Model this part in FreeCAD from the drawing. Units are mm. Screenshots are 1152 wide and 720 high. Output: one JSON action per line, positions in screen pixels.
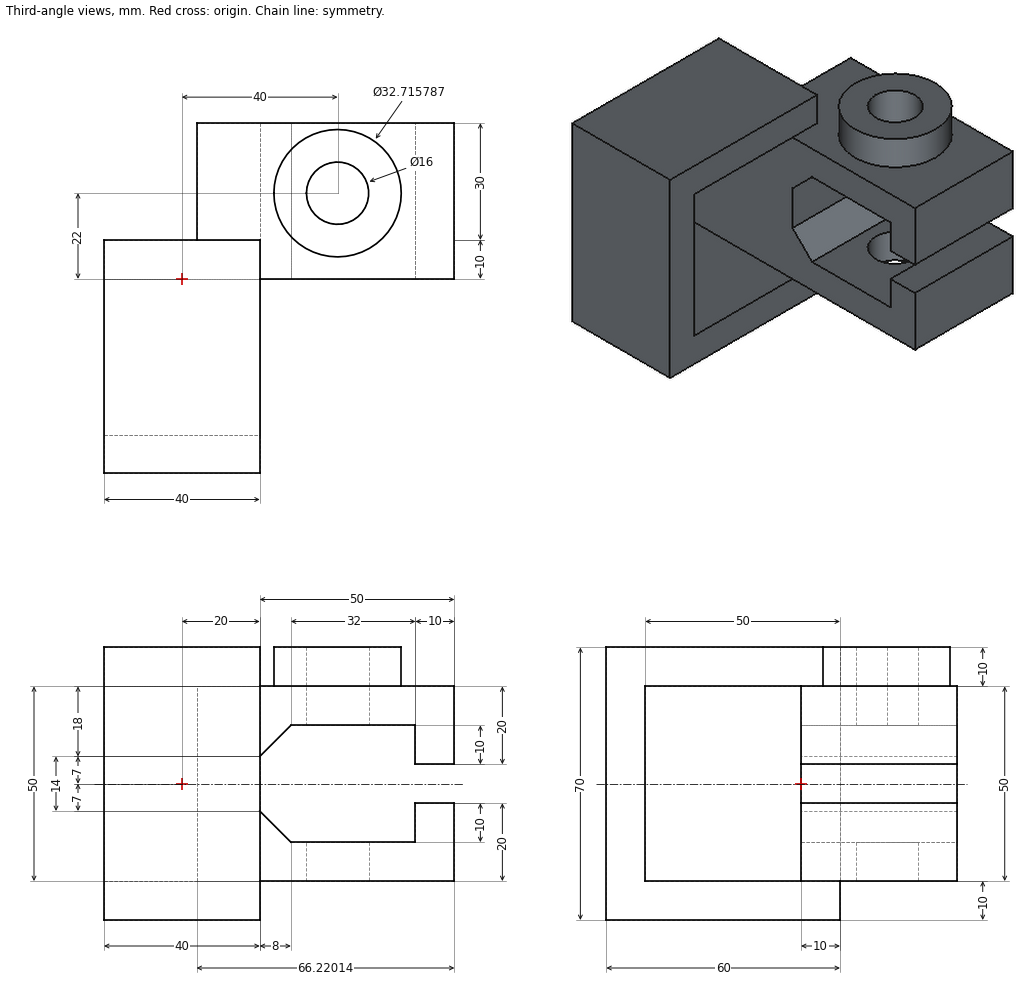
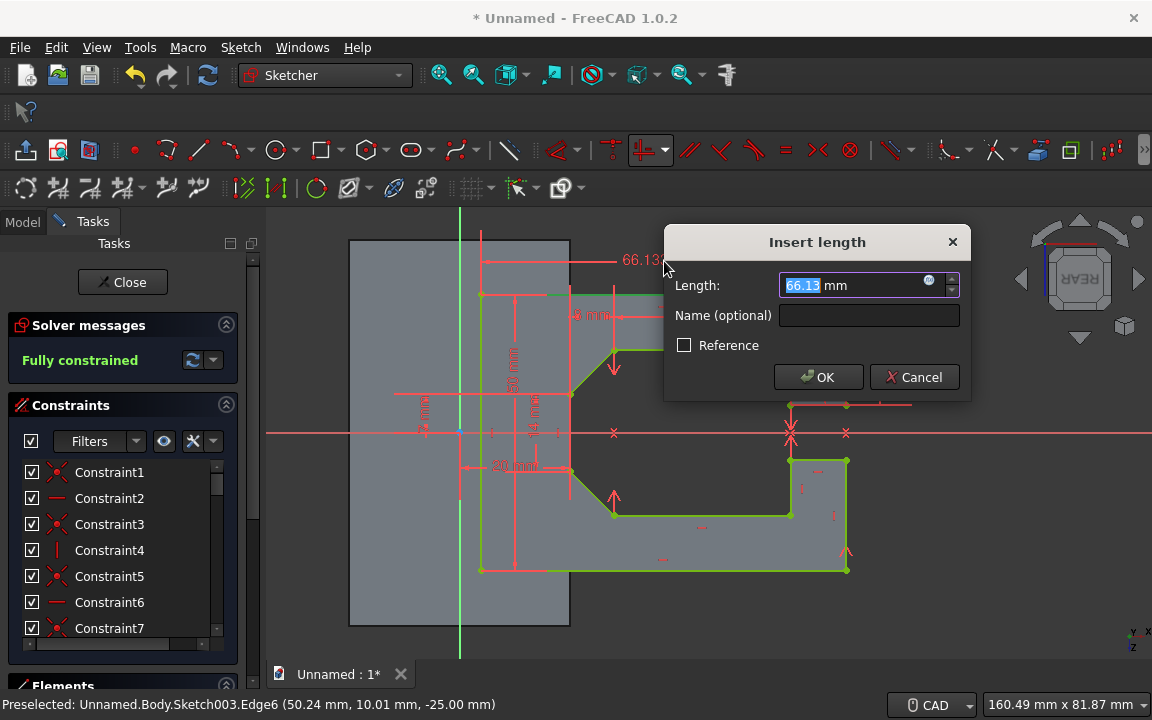
{"action": "type", "text": "66.22014"}
{"action": "key", "text": "Return"}
{"action": "key", "text": "Escape"}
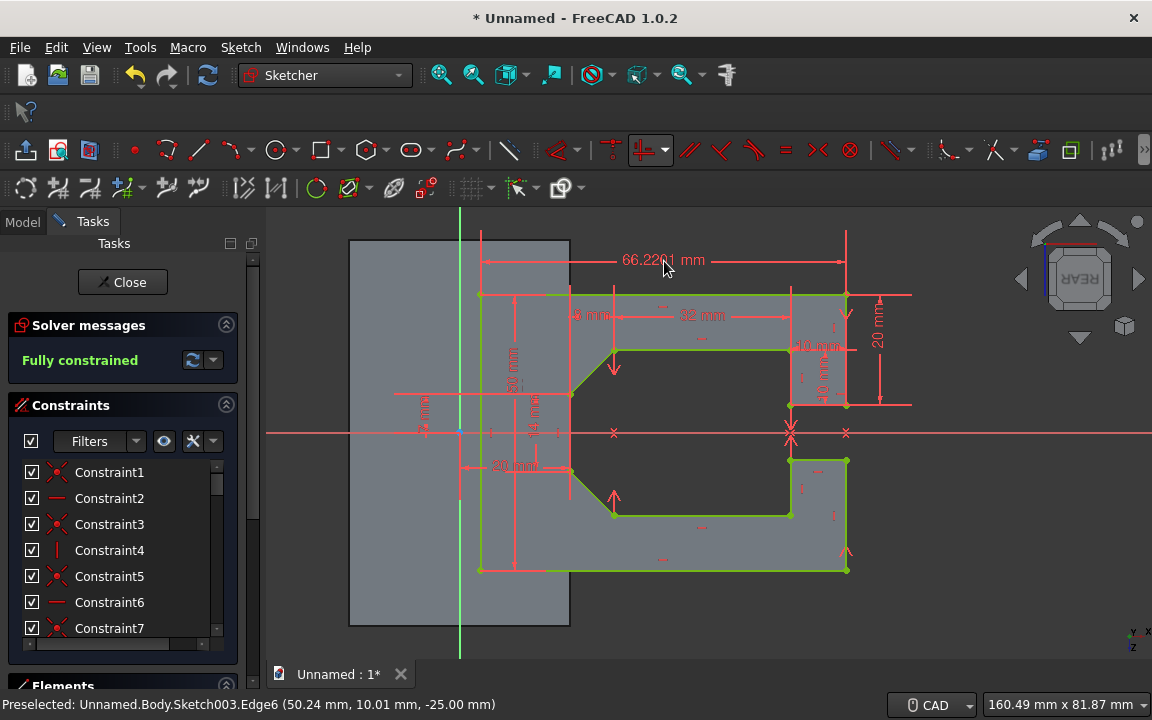
{"action": "left_click", "coordinate": [123, 282]}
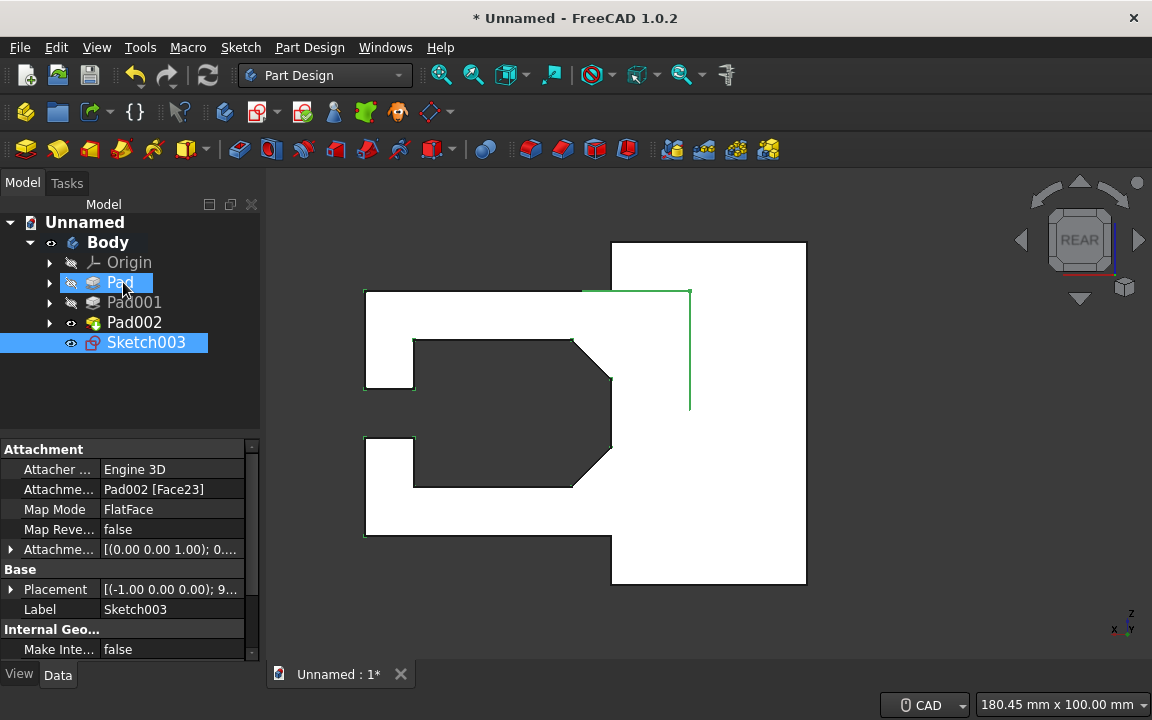
{"action": "left_click", "coordinate": [26, 150]}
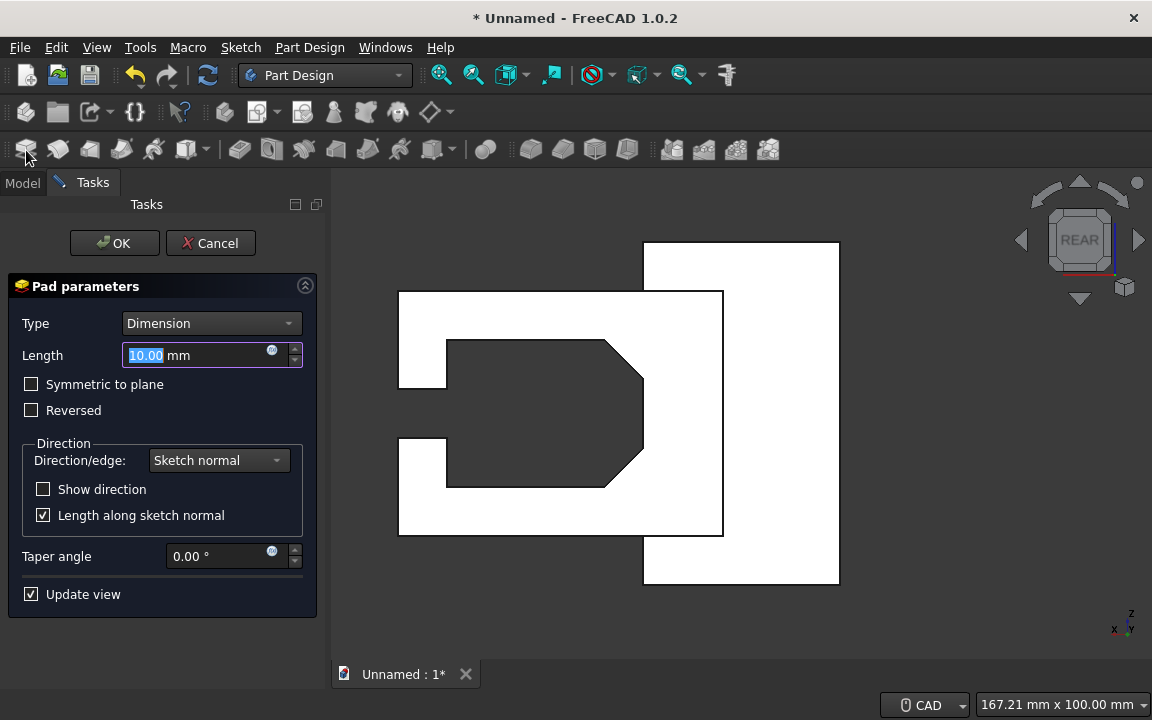
{"action": "type", "text": "30"}
{"action": "key", "text": "Tab"}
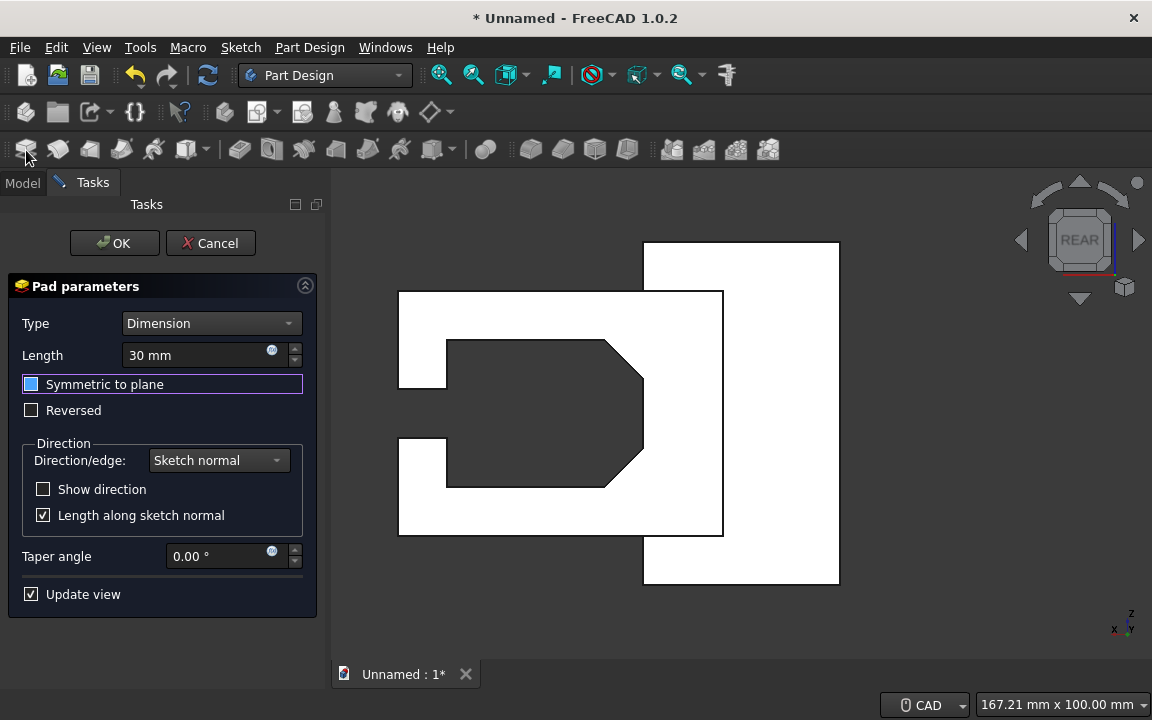
{"action": "left_click", "coordinate": [115, 243]}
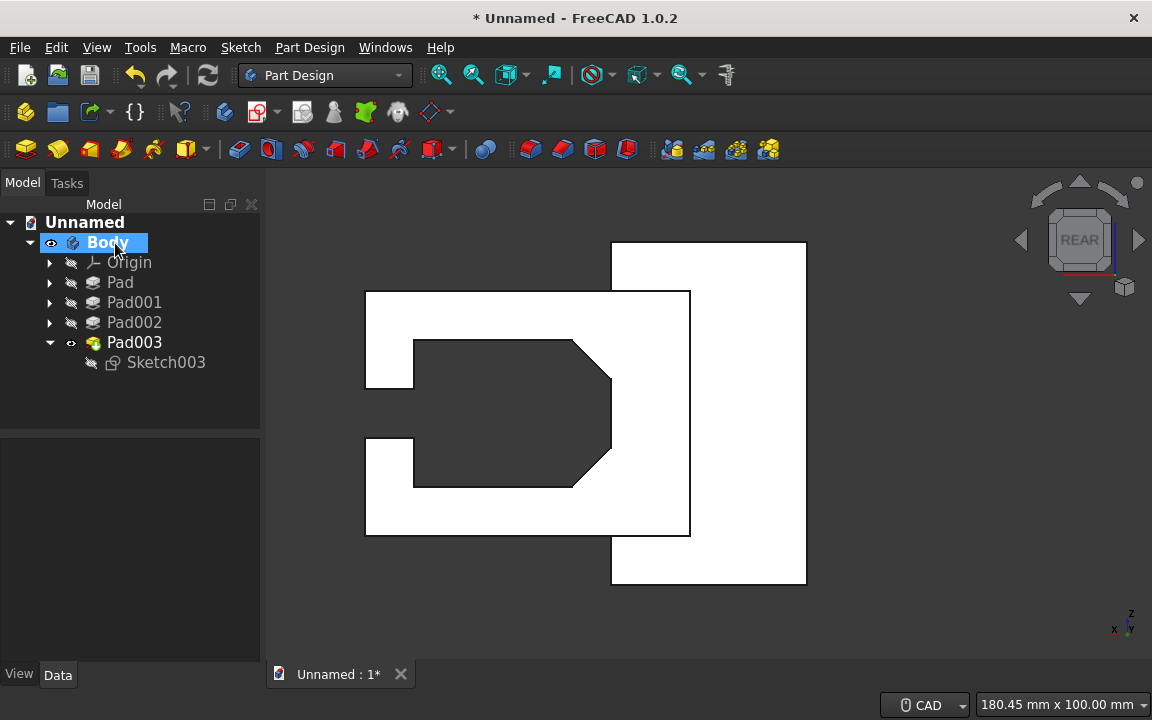
{"action": "key", "text": "5"}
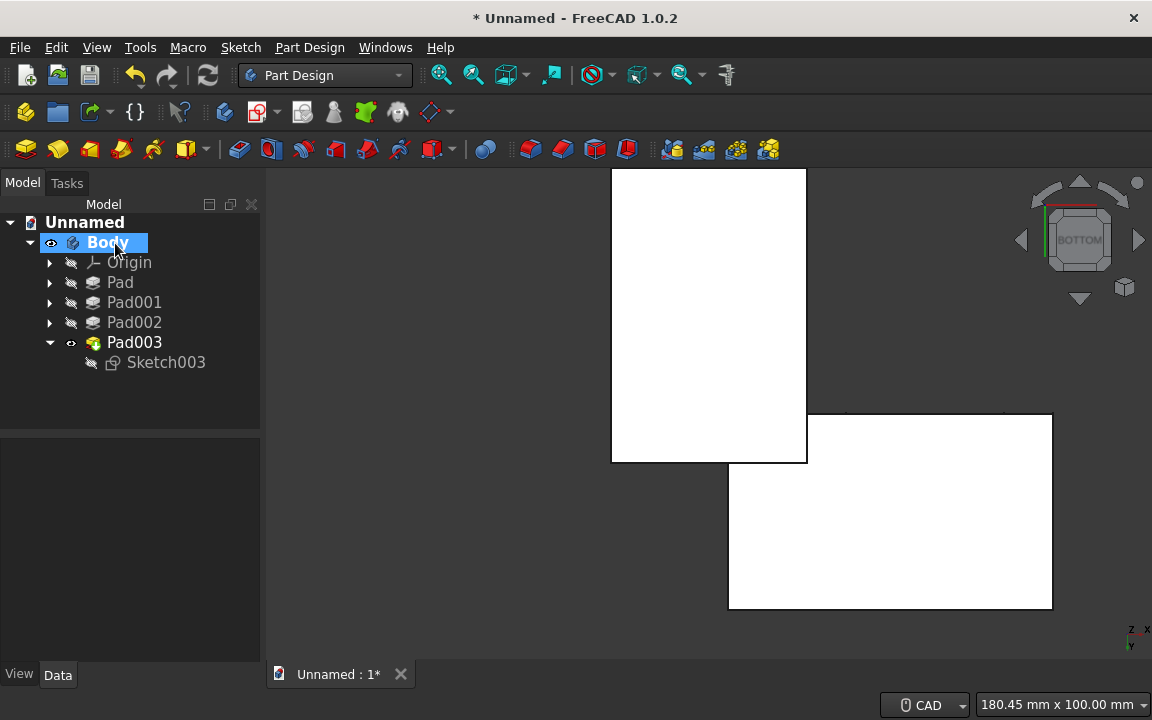
{"action": "key", "text": "v f"}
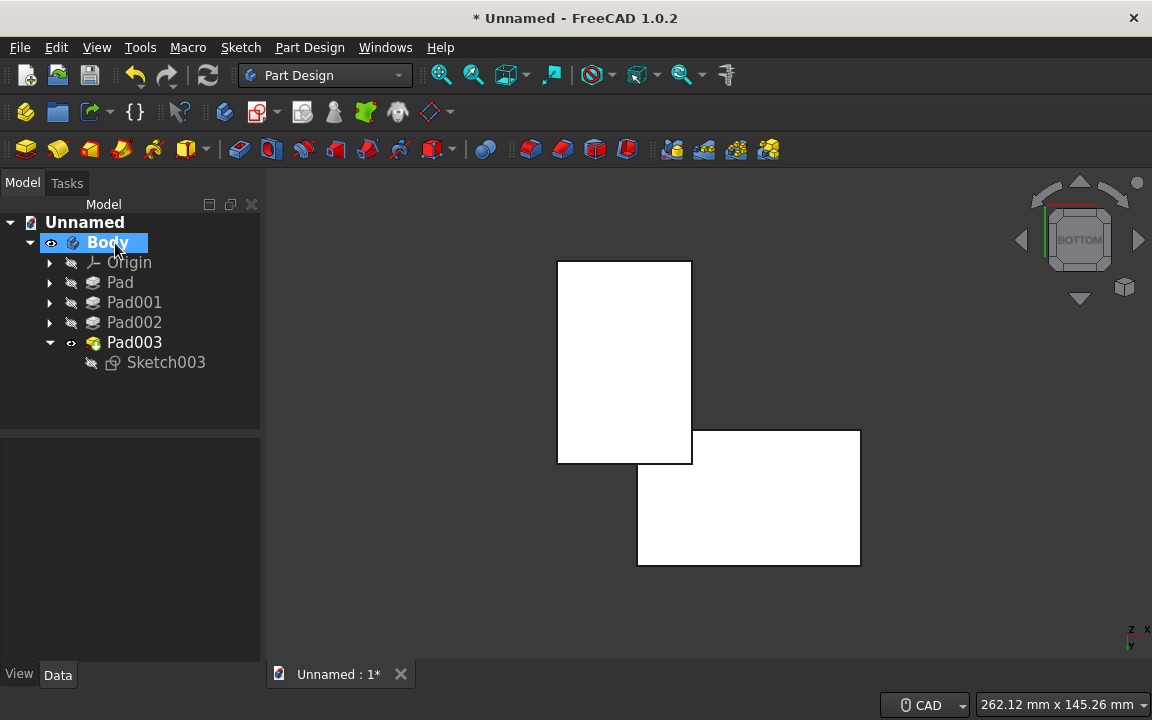
{"action": "left_click", "coordinate": [781, 497]}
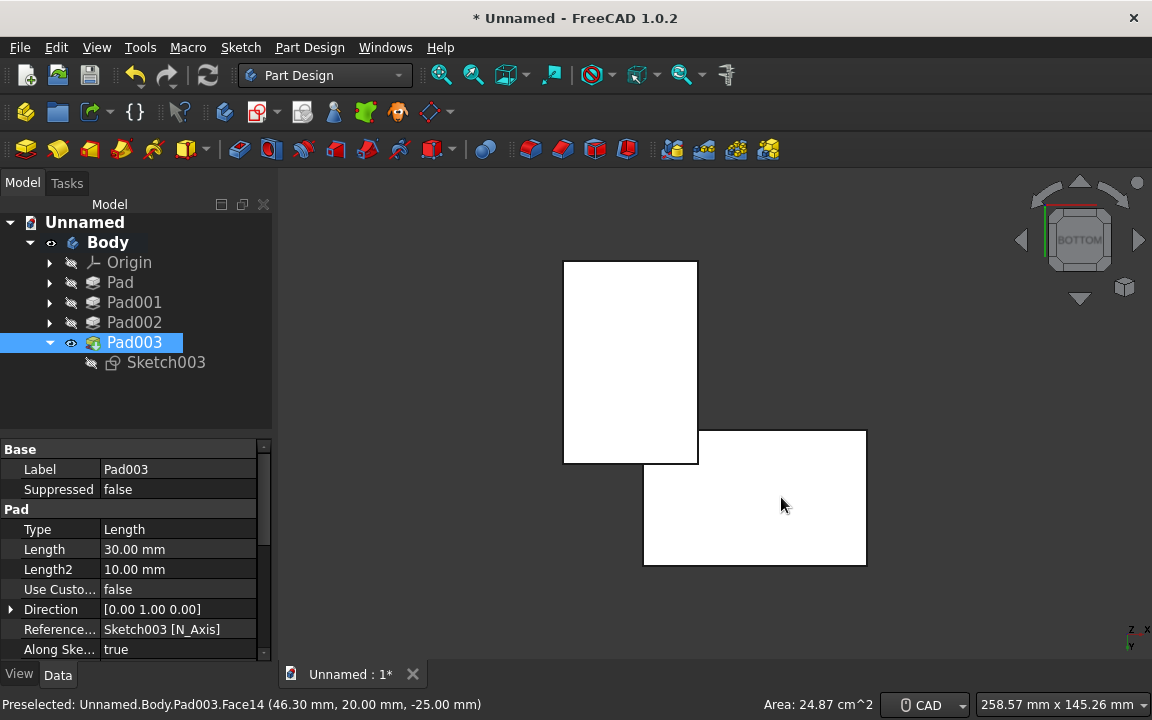
{"action": "left_click", "coordinate": [258, 112]}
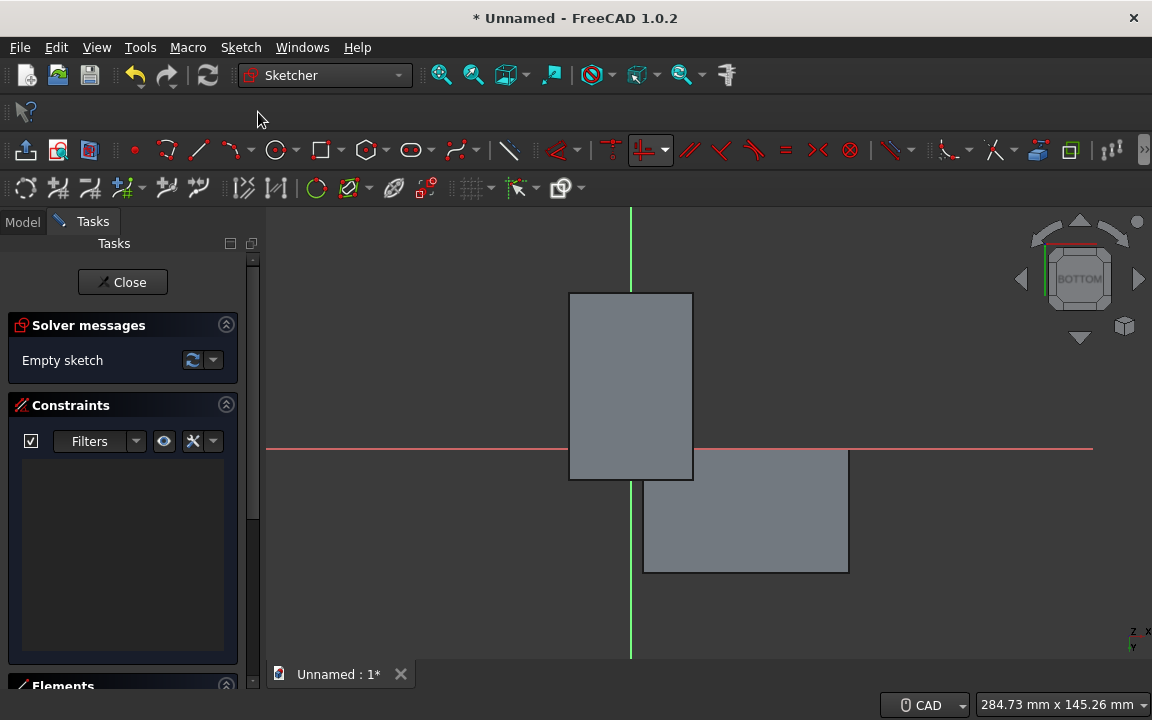
{"action": "scroll", "coordinate": [778, 534], "scroll_direction": "up", "scroll_amount": 9}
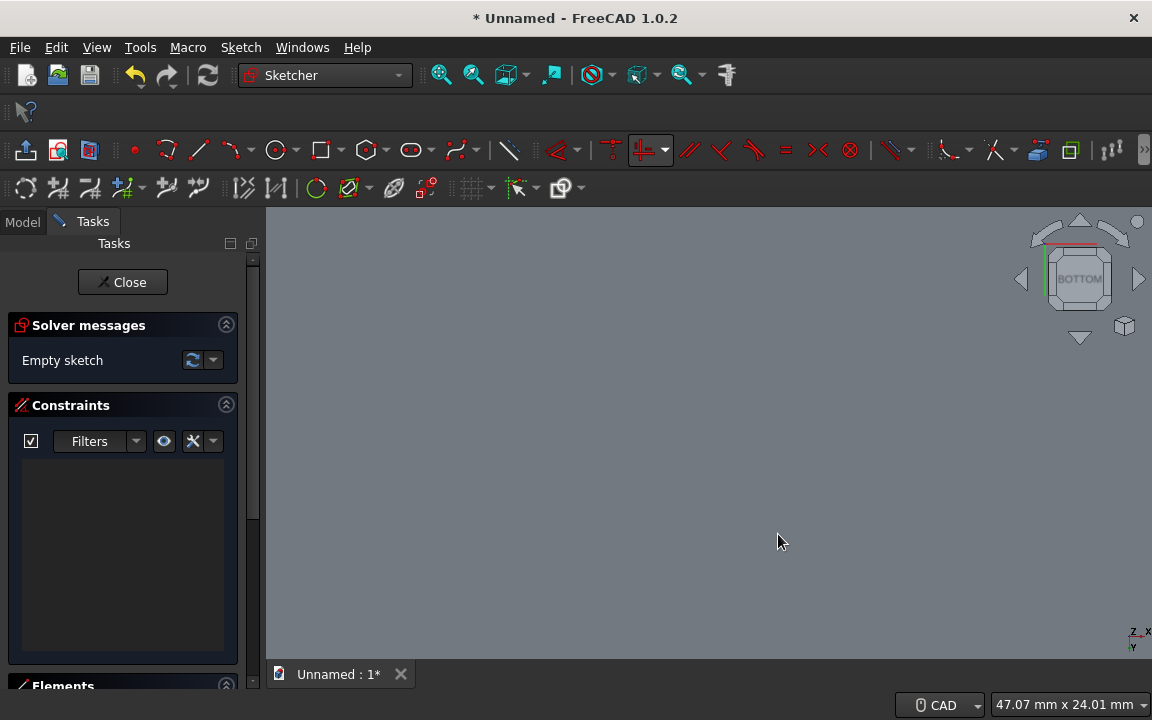
{"action": "key", "text": "g c"}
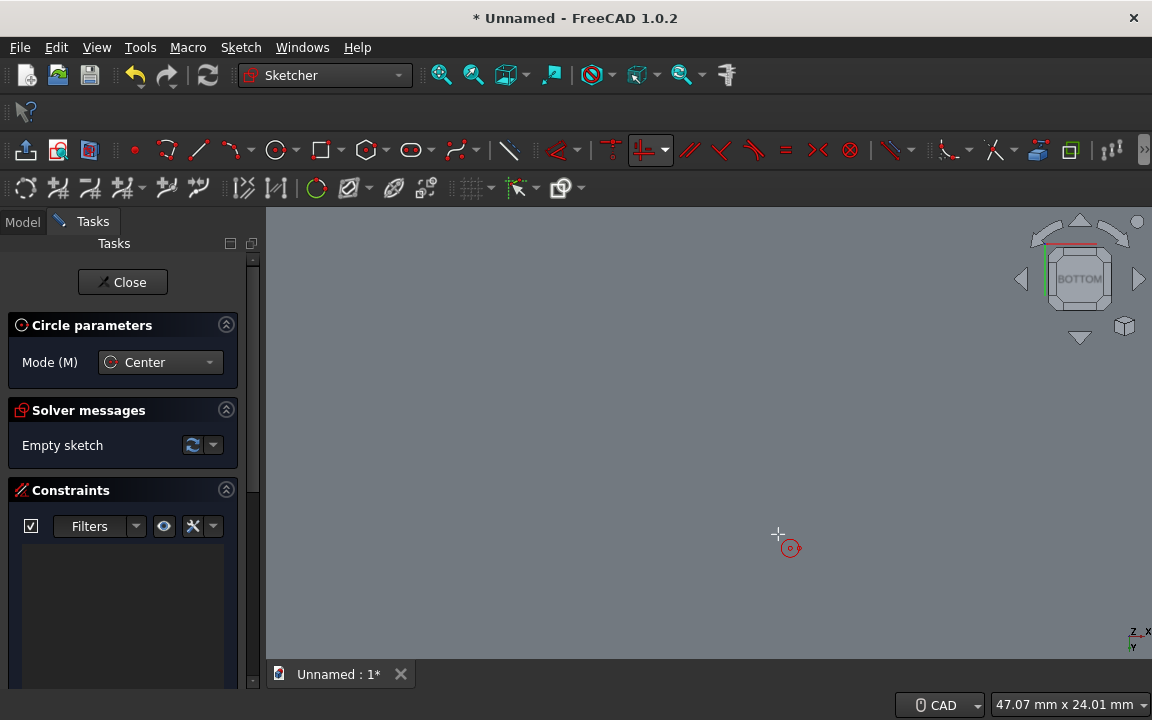
{"action": "left_click", "coordinate": [640, 428]}
{"action": "left_click", "coordinate": [747, 321]}
{"action": "key", "text": "Escape"}